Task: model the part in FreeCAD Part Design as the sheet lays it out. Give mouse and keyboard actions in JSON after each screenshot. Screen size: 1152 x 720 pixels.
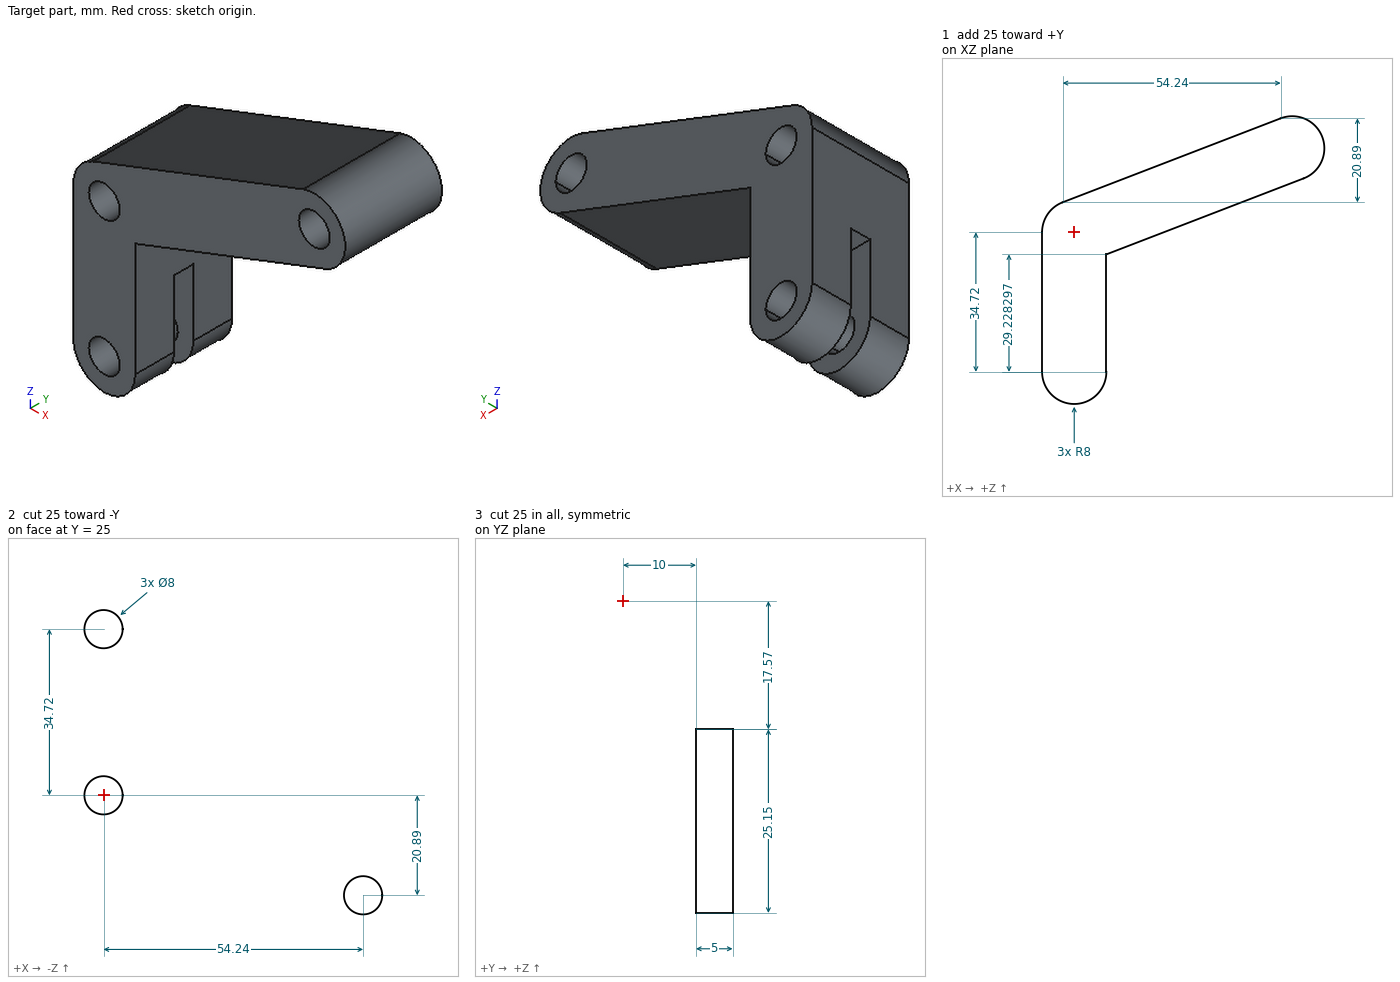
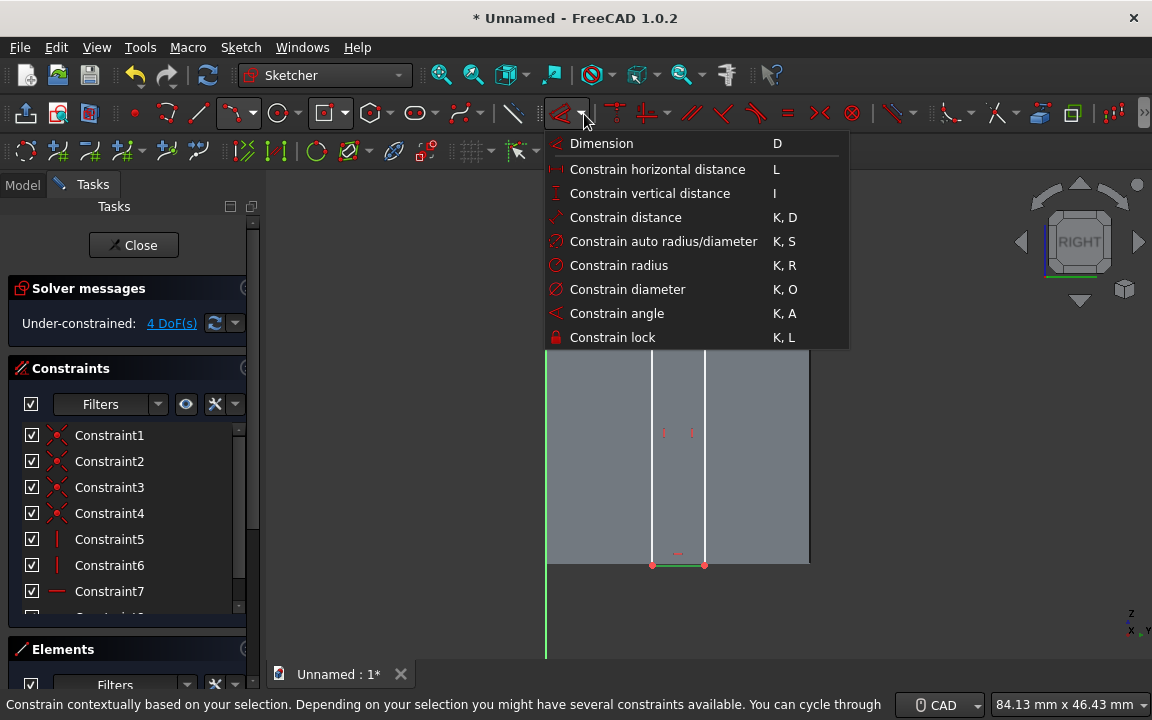
{"action": "left_click", "coordinate": [697, 169]}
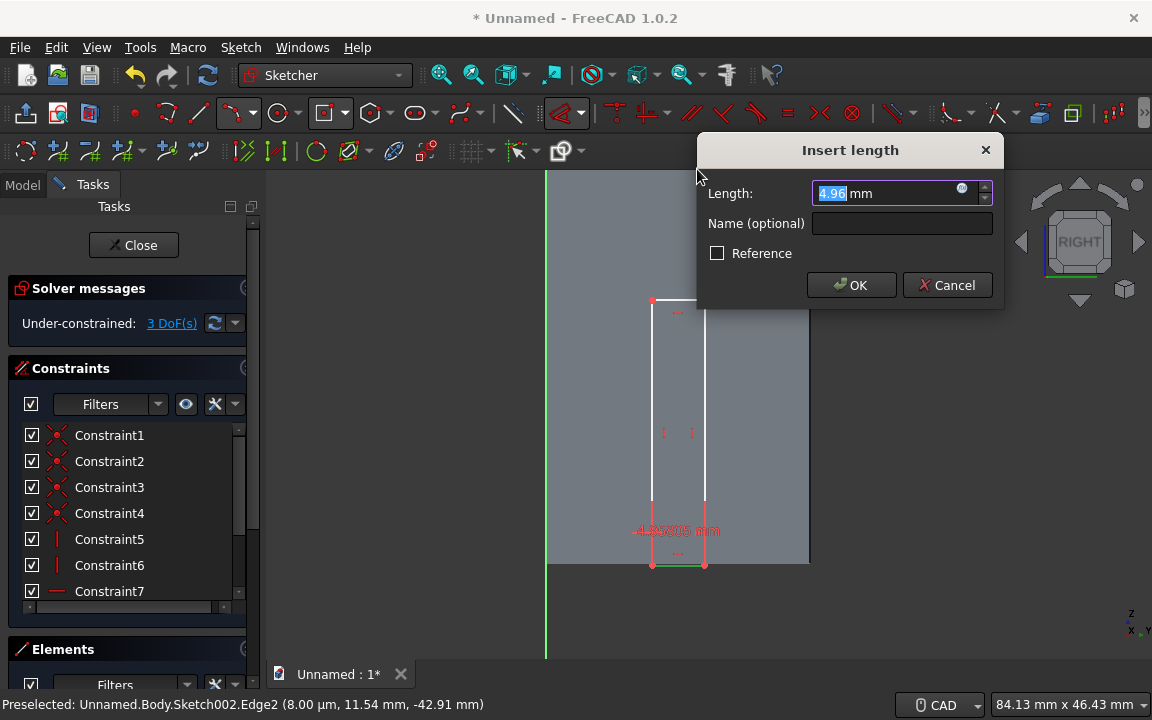
{"action": "type", "text": "5"}
{"action": "key", "text": "Return"}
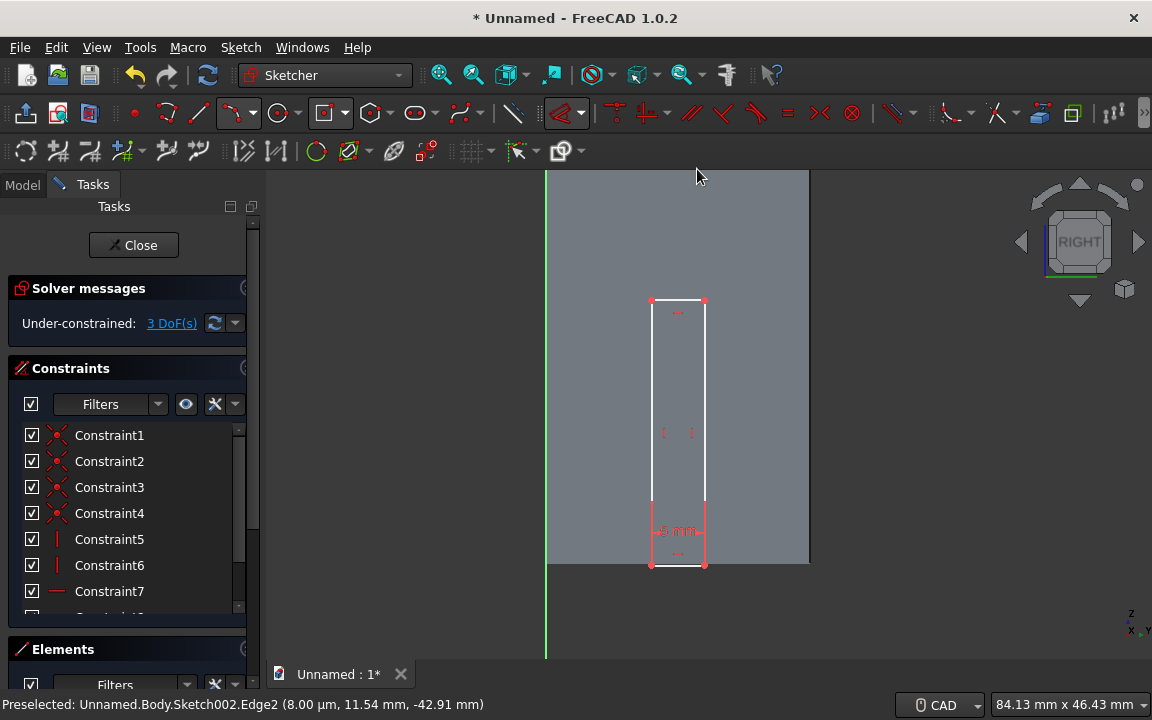
{"action": "left_click", "coordinate": [652, 300]}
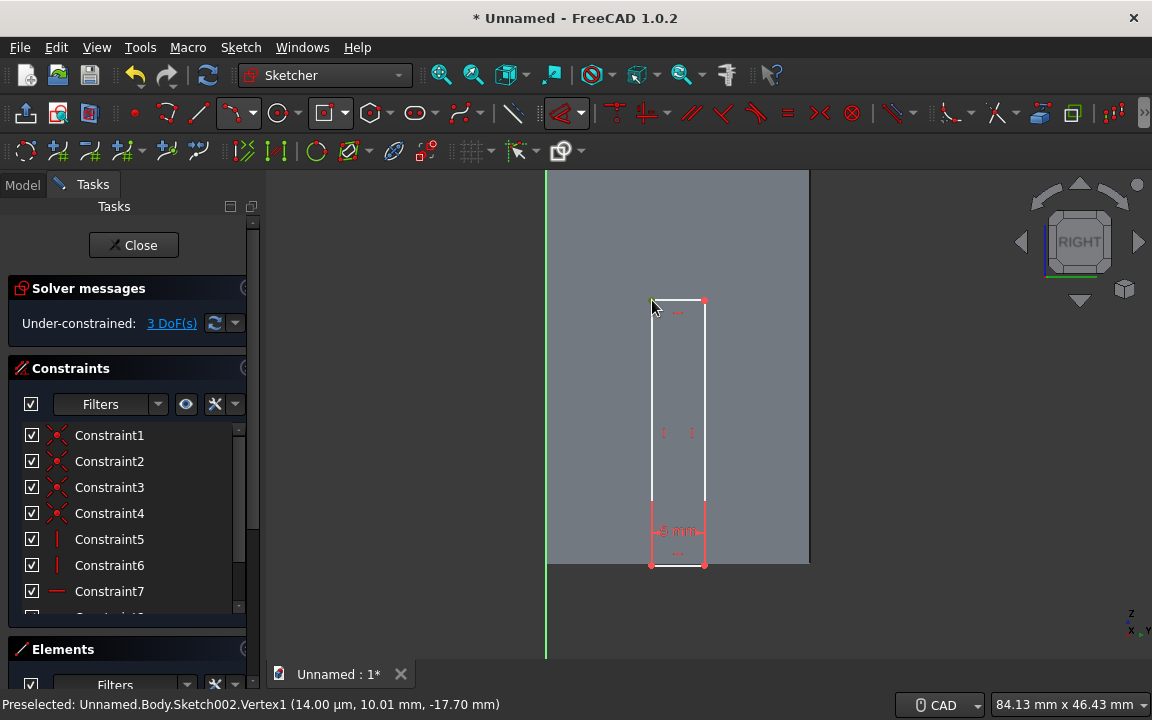
{"action": "left_click", "coordinate": [584, 114]}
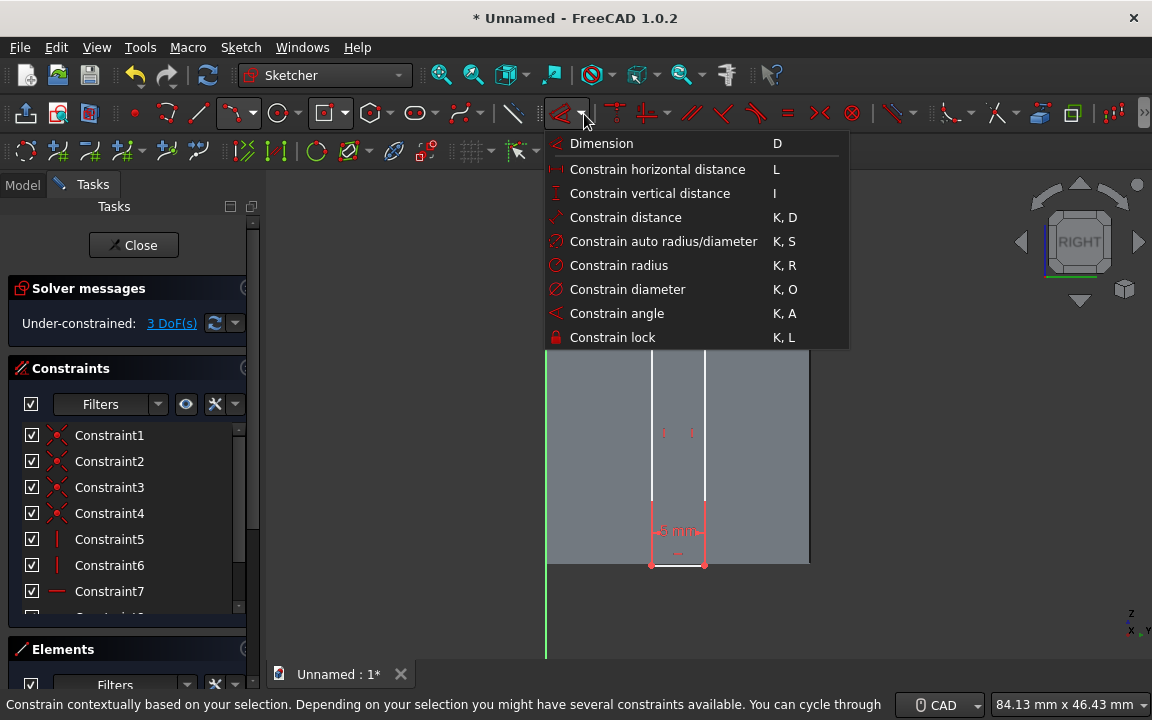
{"action": "left_click", "coordinate": [697, 169]}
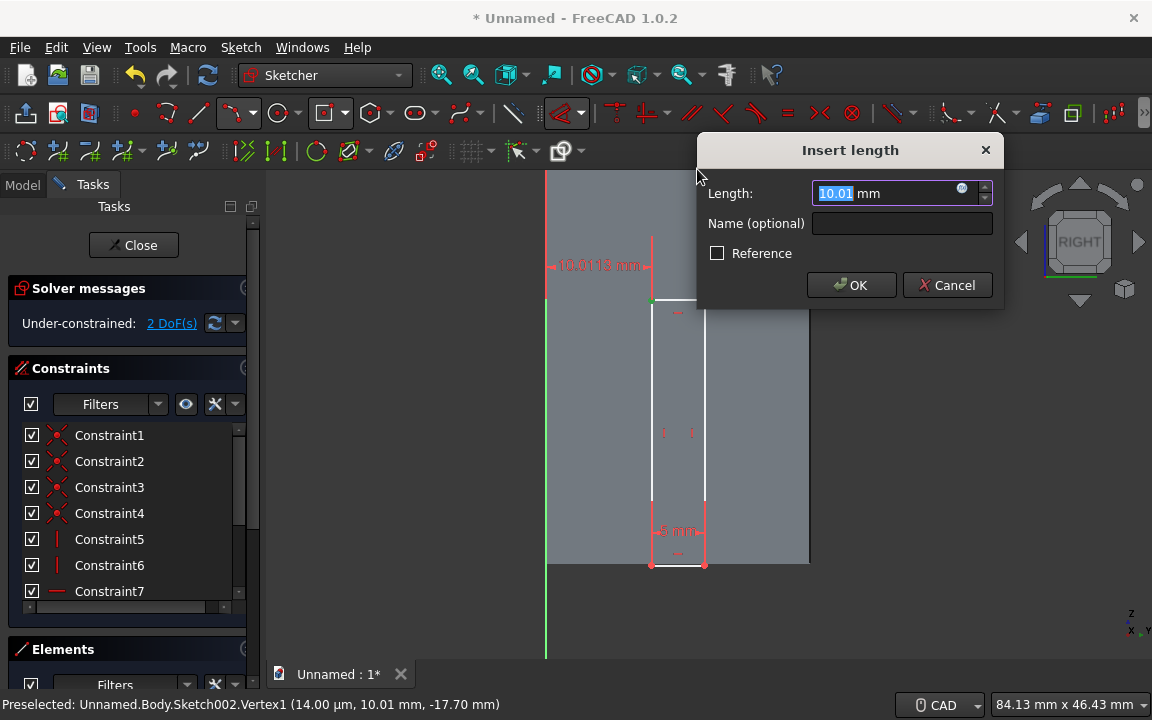
{"action": "type", "text": "10"}
{"action": "key", "text": "Return"}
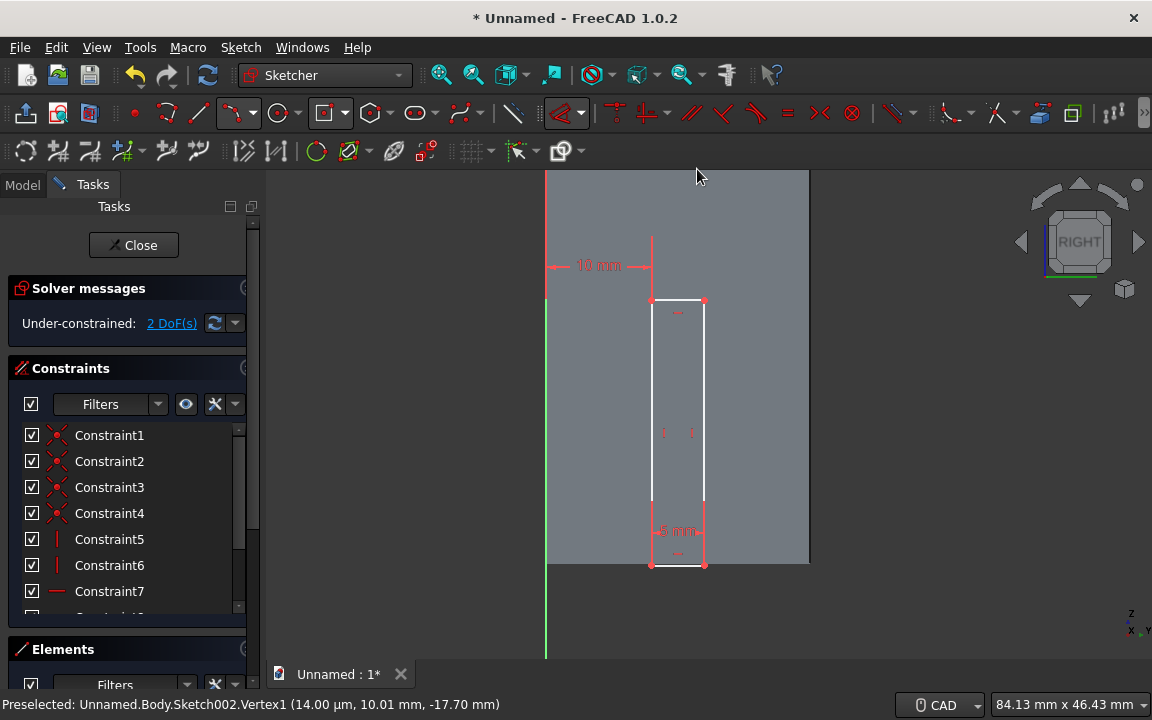
{"action": "left_click", "coordinate": [652, 380]}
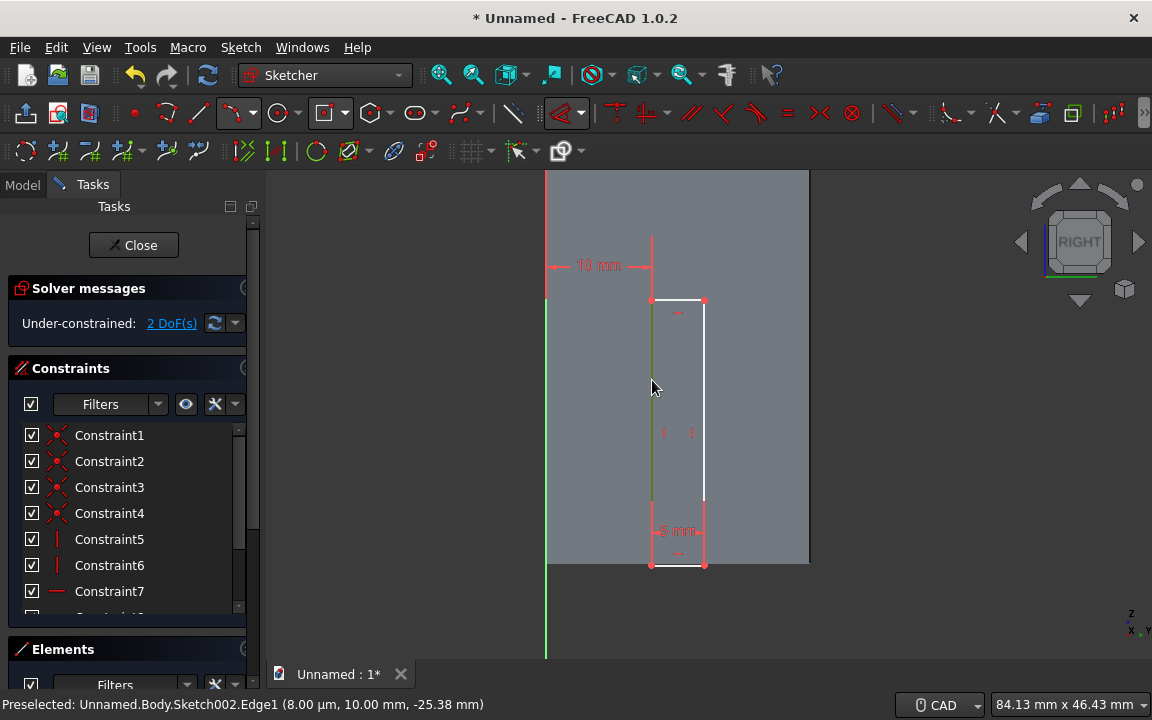
{"action": "key", "text": "i"}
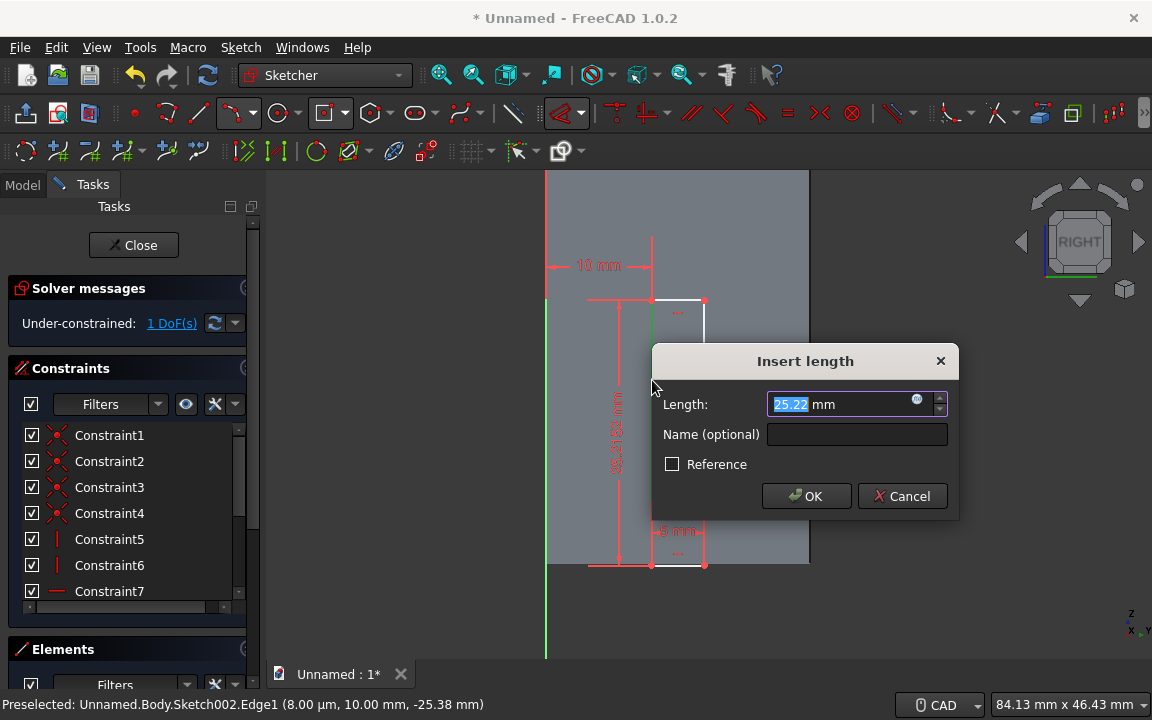
{"action": "type", "text": "25.15"}
{"action": "key", "text": "Return"}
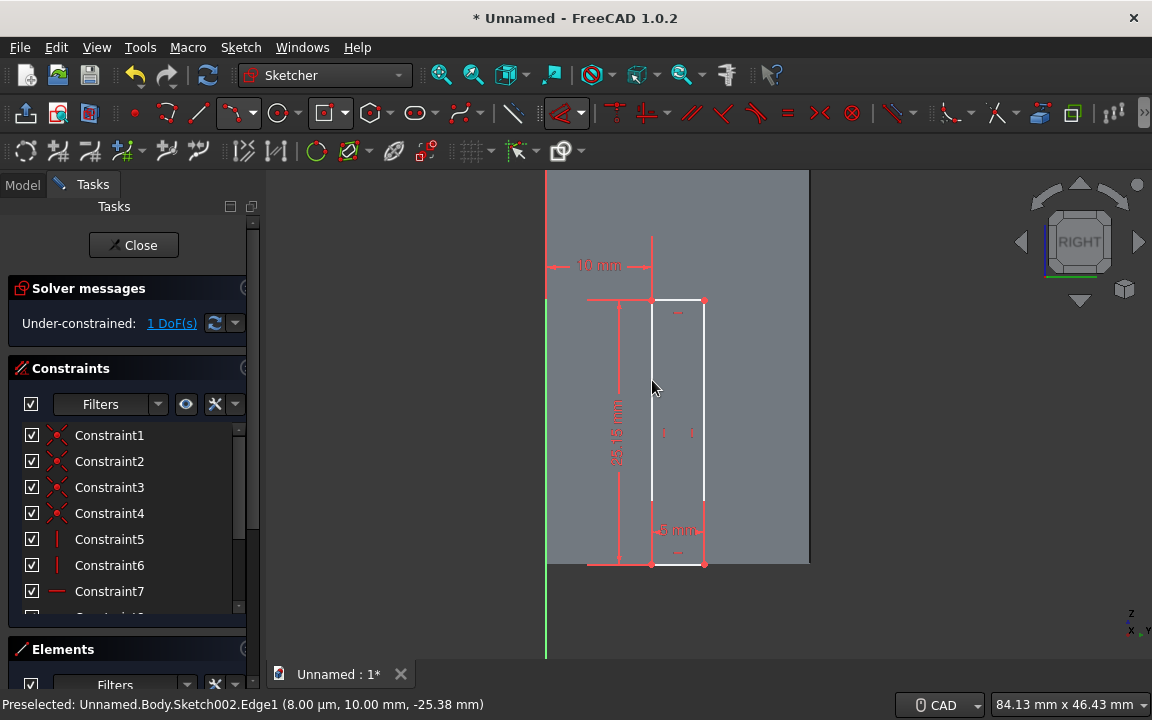
{"action": "left_click", "coordinate": [652, 300]}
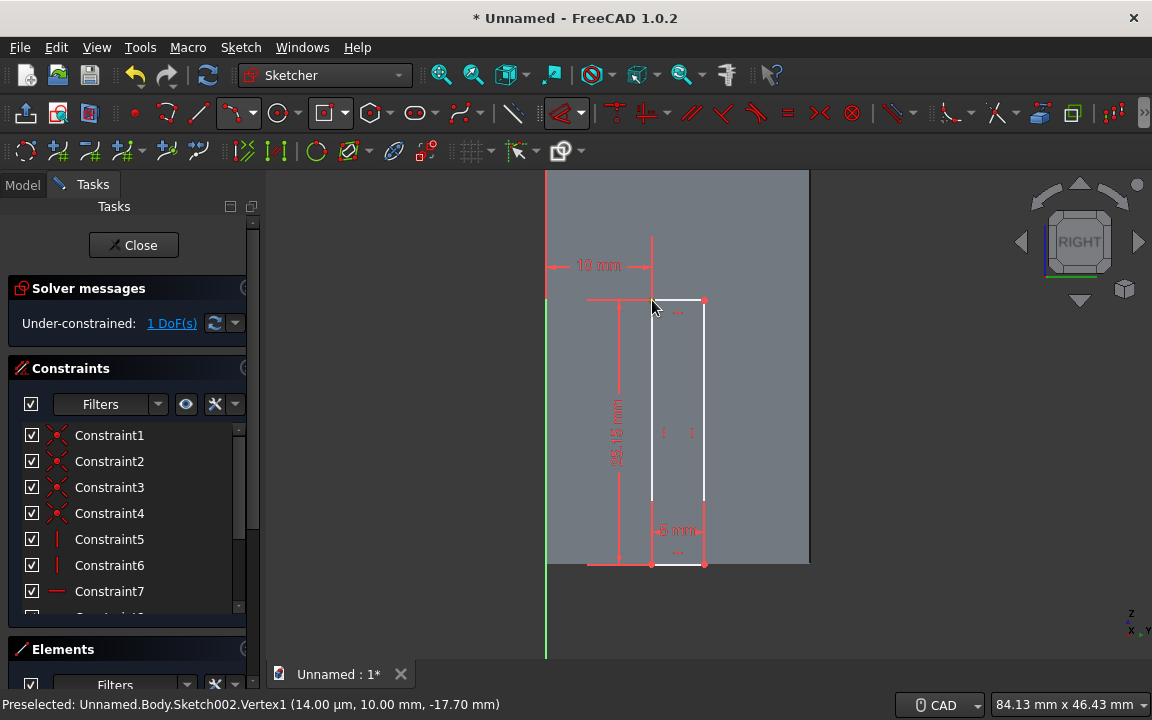
{"action": "key", "text": "i"}